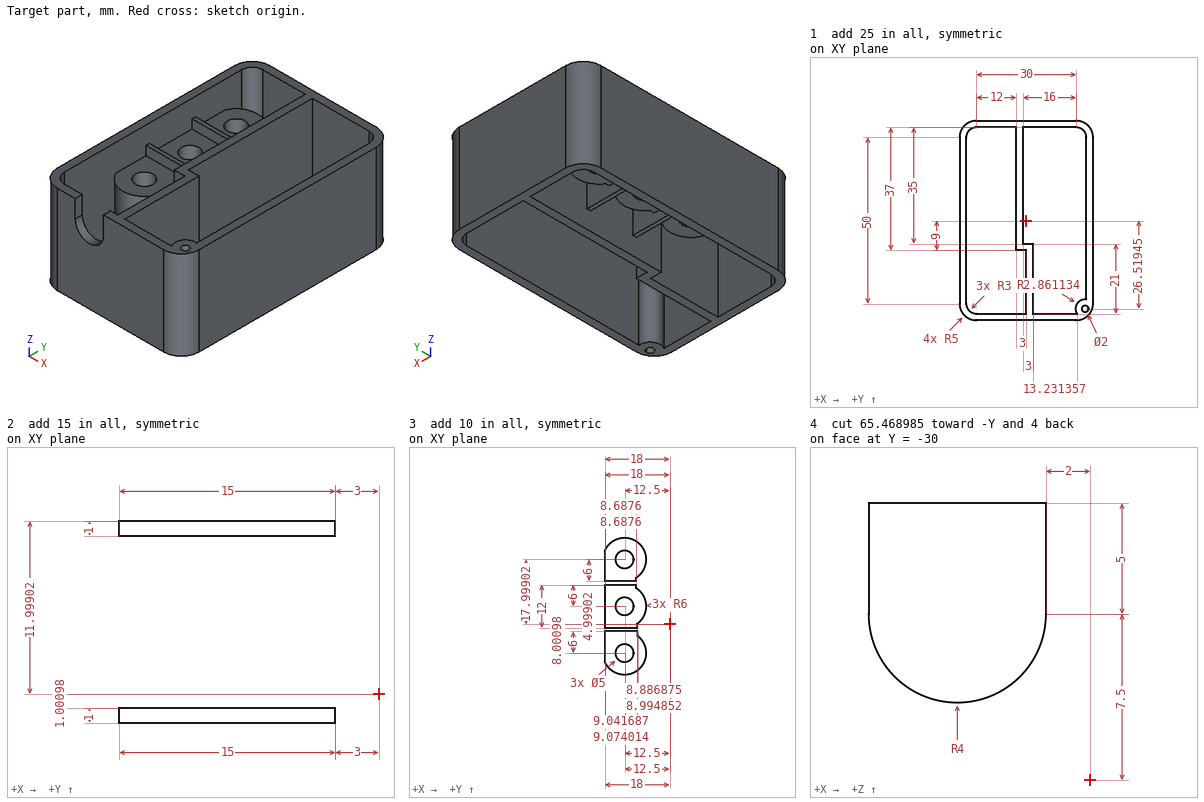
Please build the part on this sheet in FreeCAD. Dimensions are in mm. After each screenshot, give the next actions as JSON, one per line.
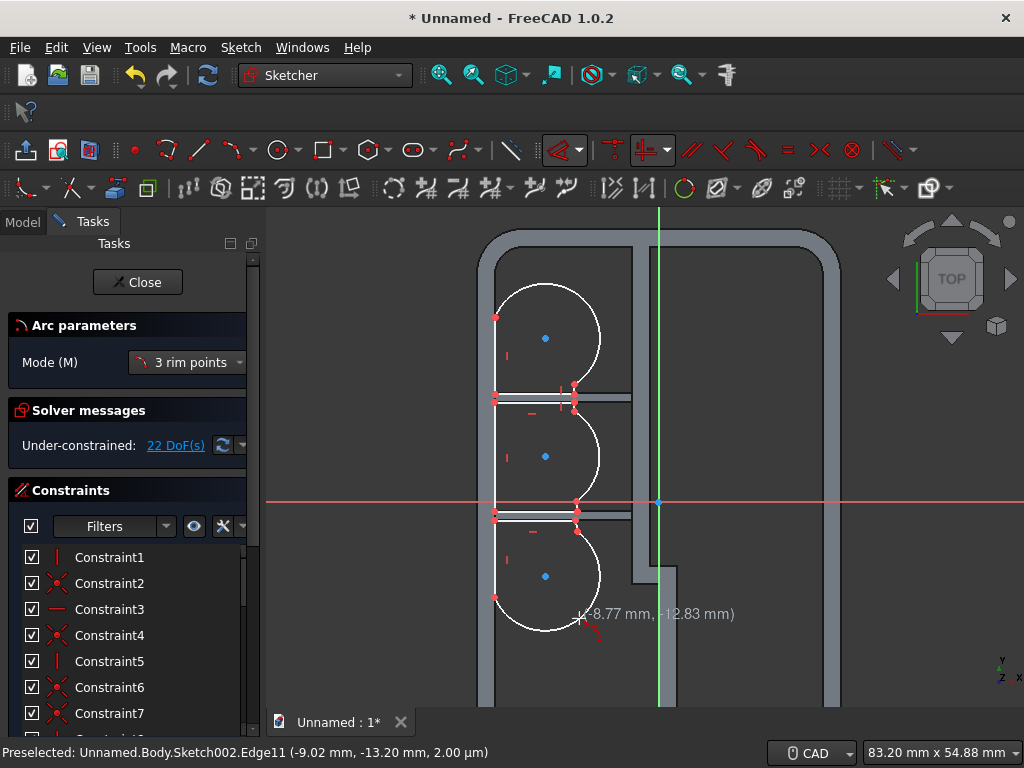
{"action": "left_click", "coordinate": [278, 150]}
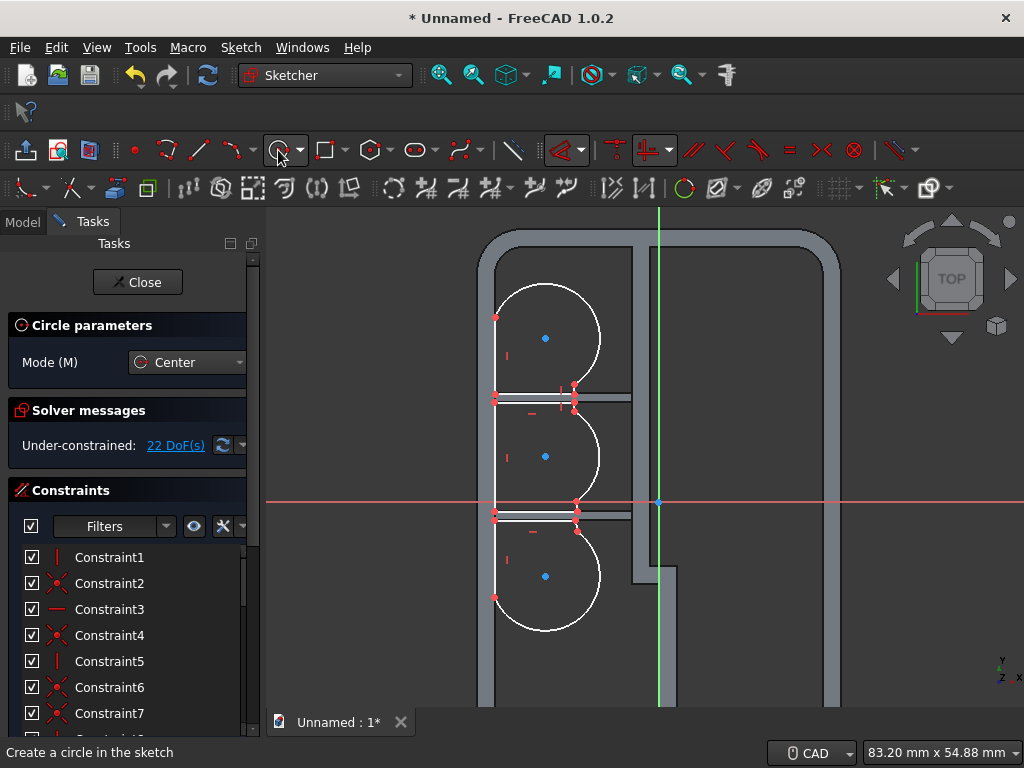
{"action": "left_click", "coordinate": [545, 338]}
{"action": "left_click", "coordinate": [561, 322]}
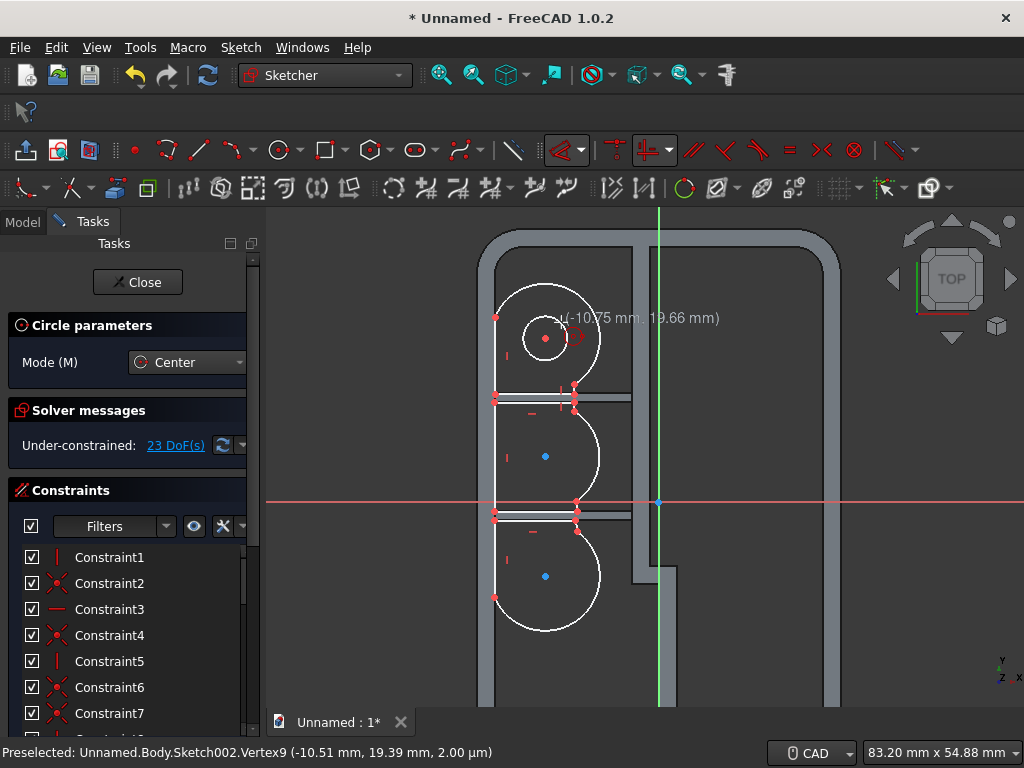
{"action": "left_click", "coordinate": [545, 457]}
{"action": "left_click", "coordinate": [561, 440]}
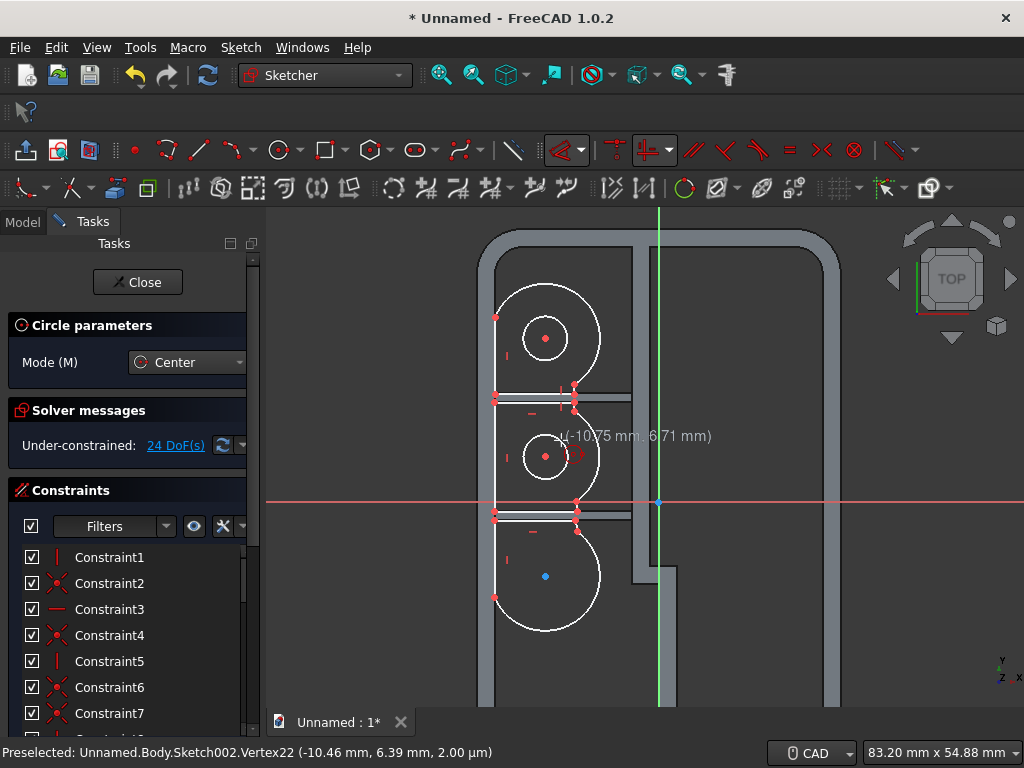
{"action": "left_click", "coordinate": [545, 575]}
{"action": "left_click", "coordinate": [561, 559]}
{"action": "key", "text": "Escape"}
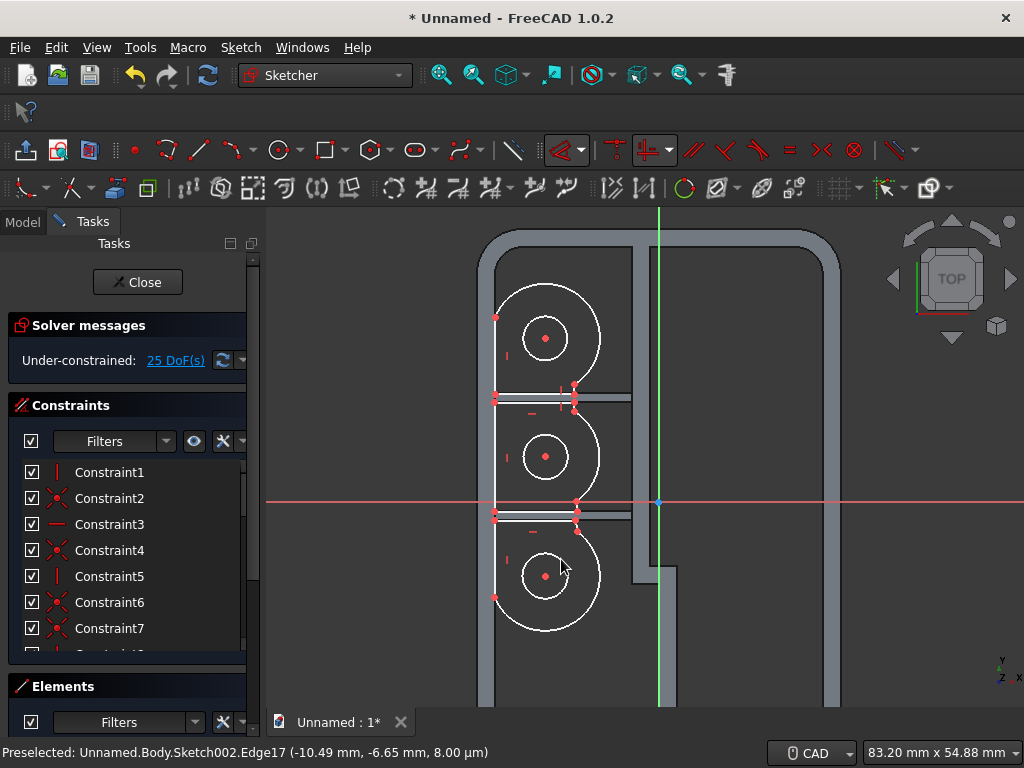
{"action": "left_click", "coordinate": [600, 332]}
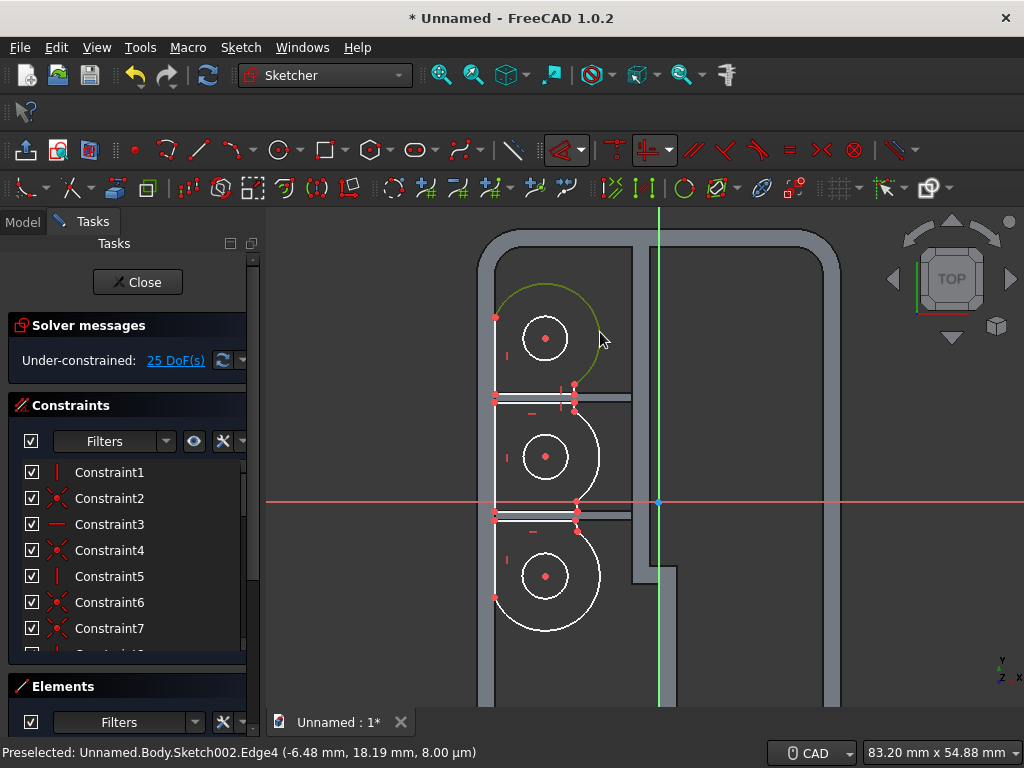
{"action": "left_click", "coordinate": [596, 476]}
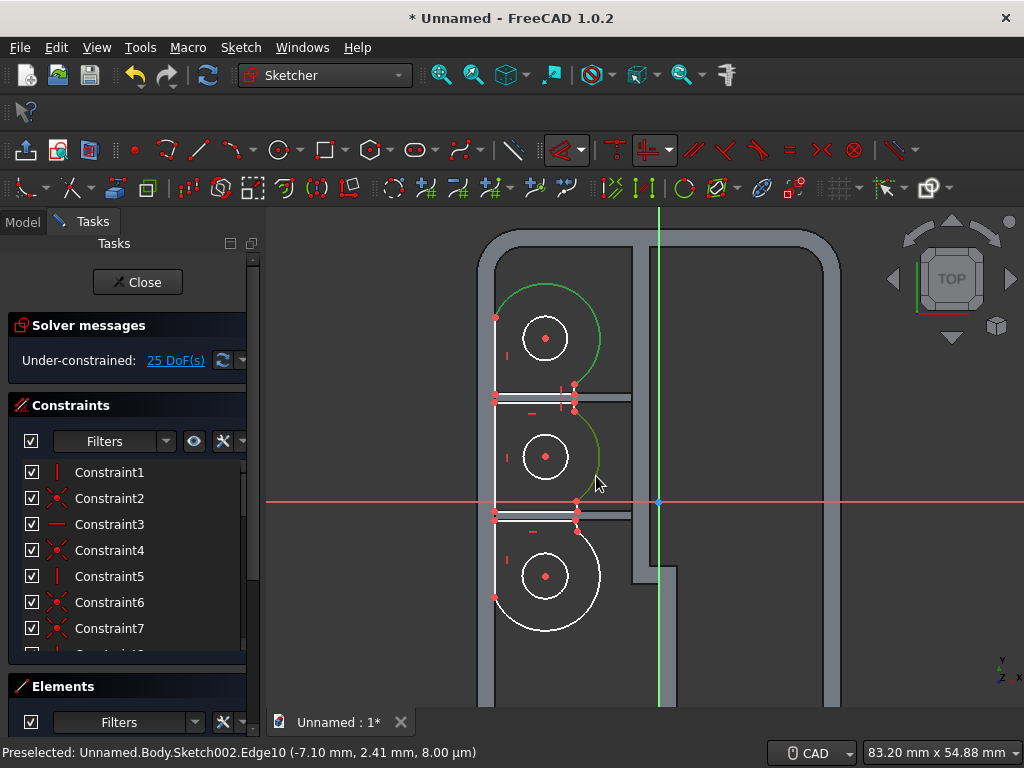
{"action": "left_click", "coordinate": [542, 631]}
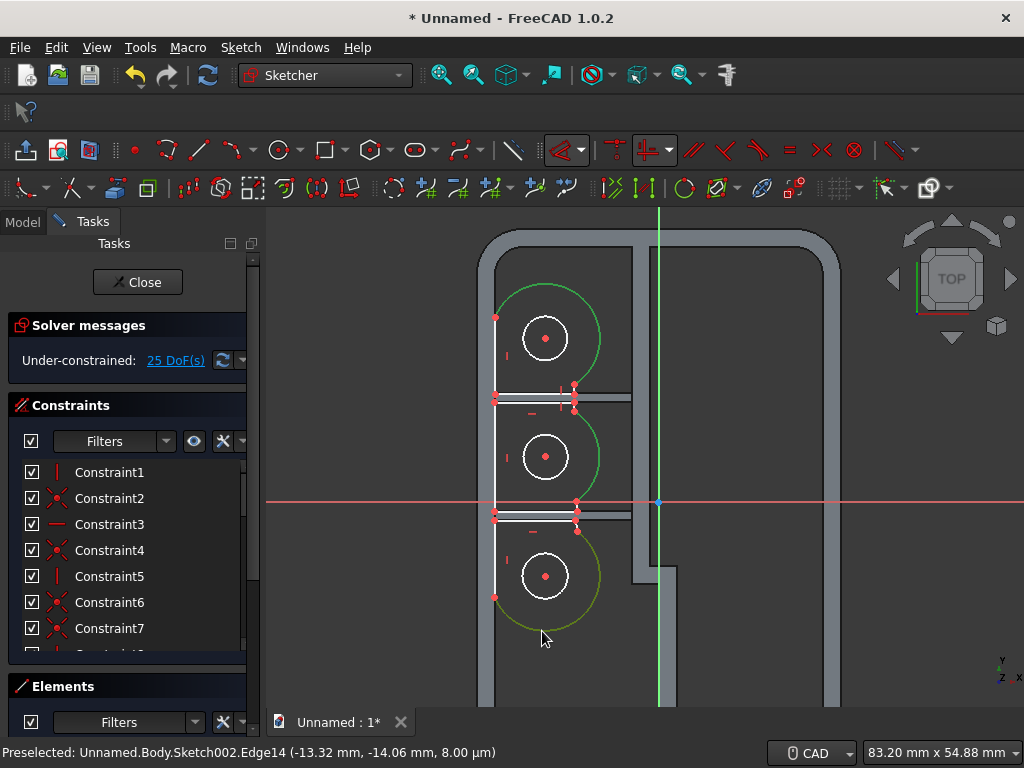
{"action": "left_click", "coordinate": [790, 150]}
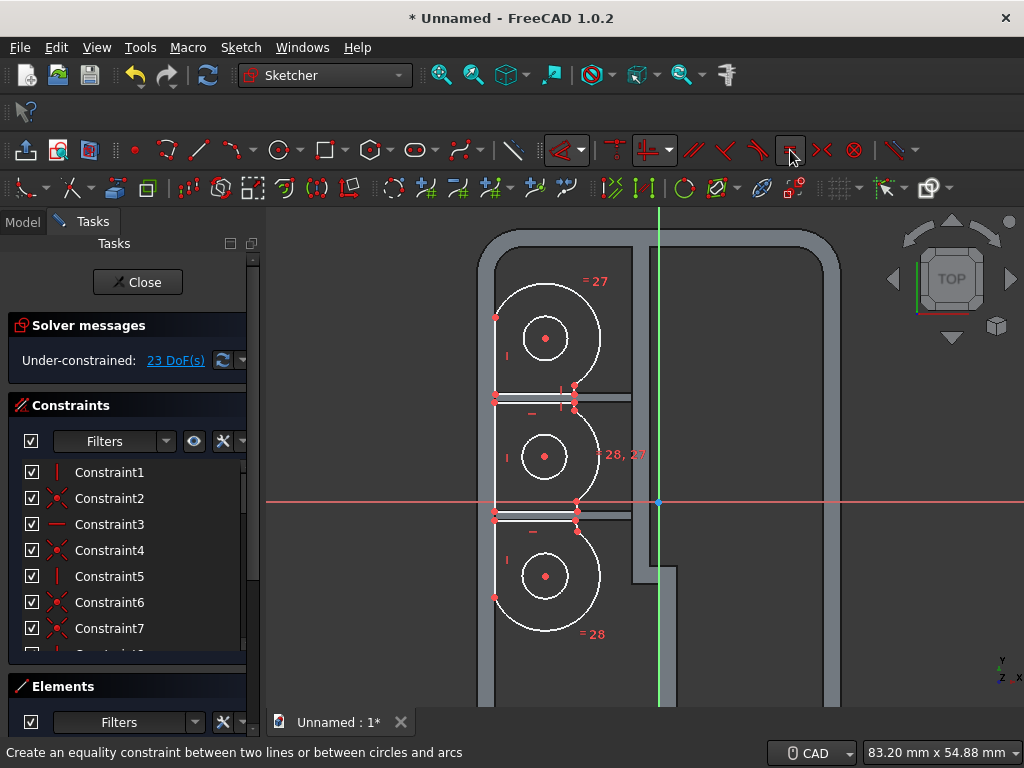
{"action": "left_click", "coordinate": [561, 323]}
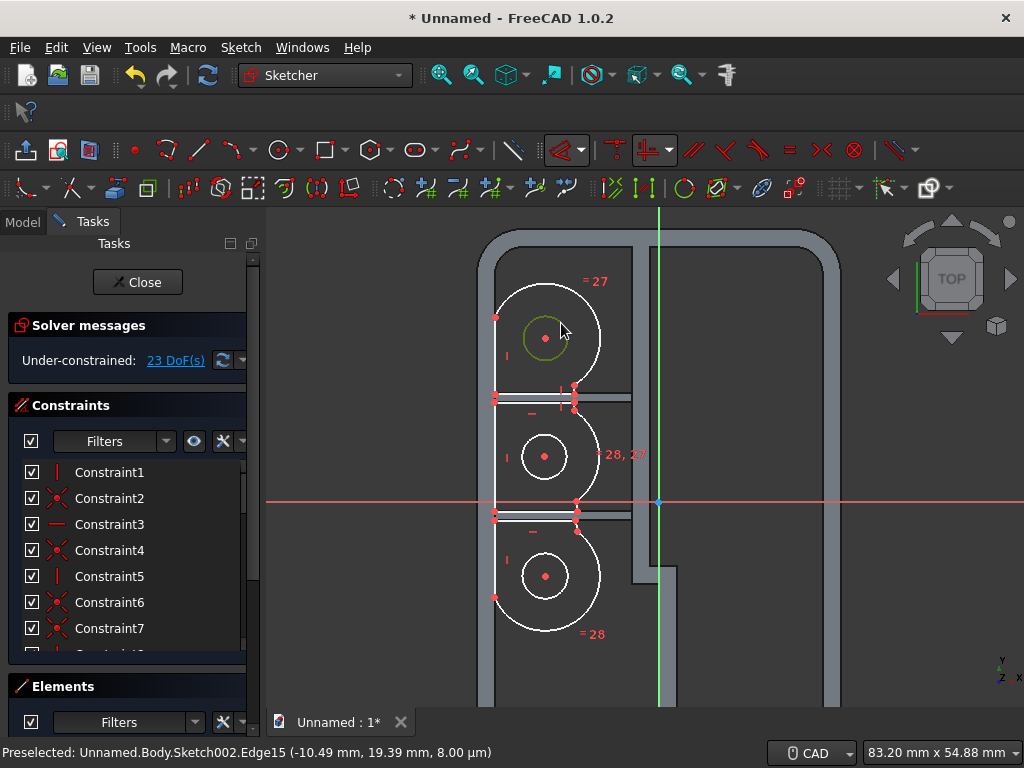
{"action": "left_click", "coordinate": [560, 441]}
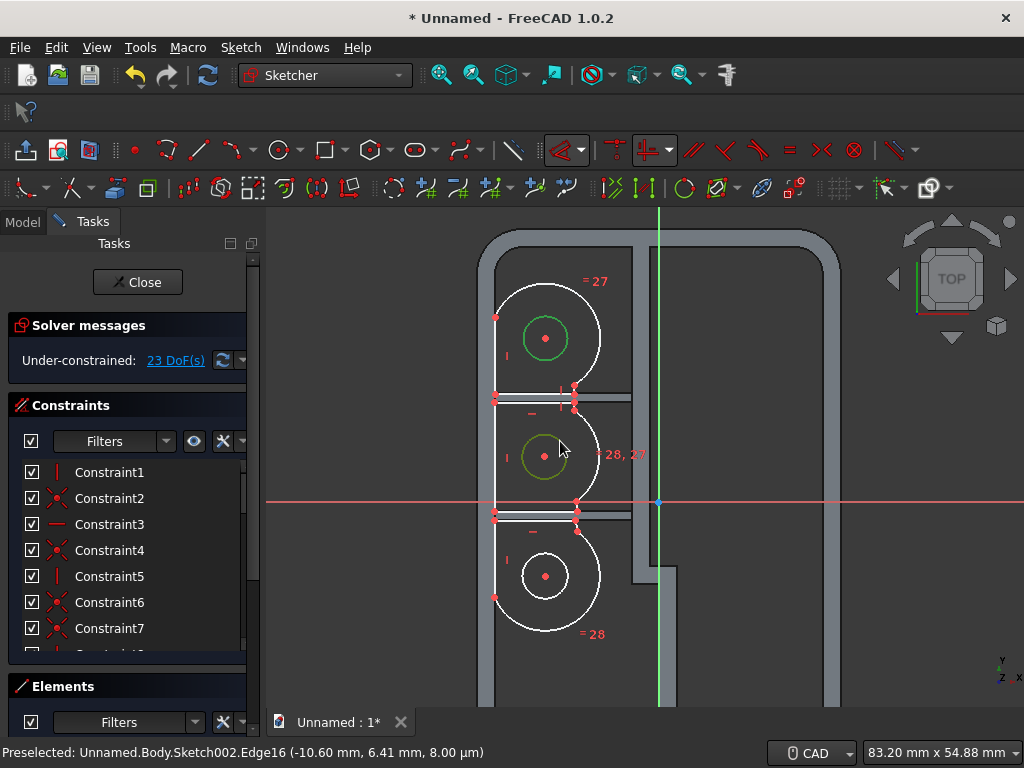
{"action": "left_click", "coordinate": [561, 560]}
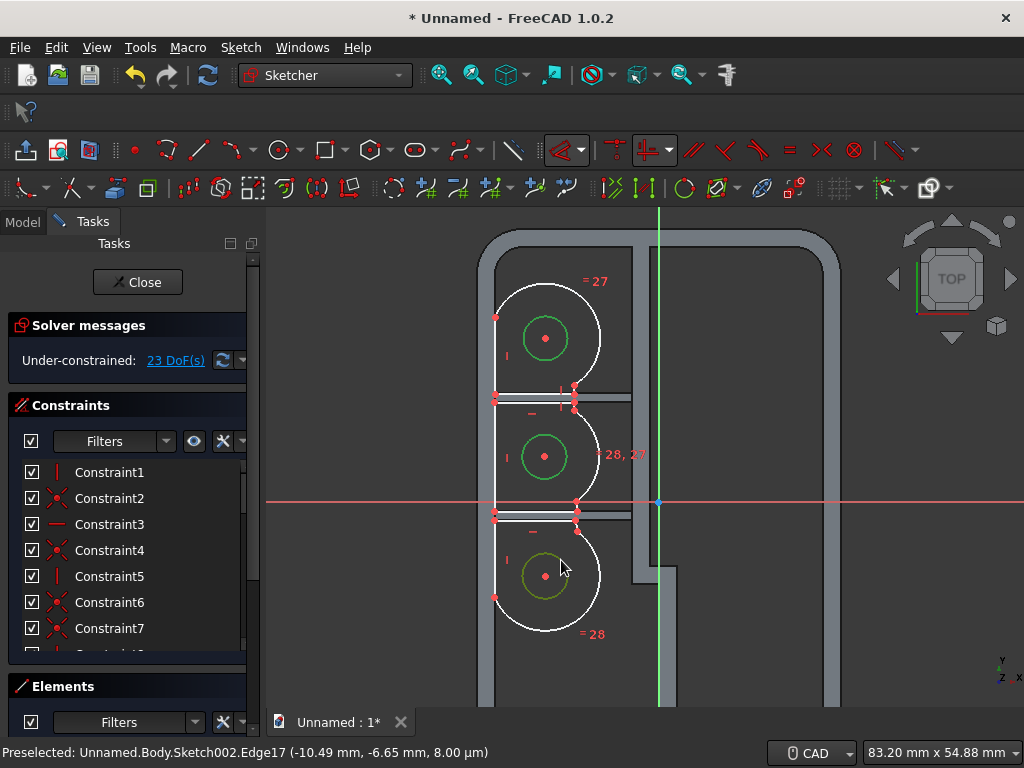
{"action": "left_click", "coordinate": [790, 150]}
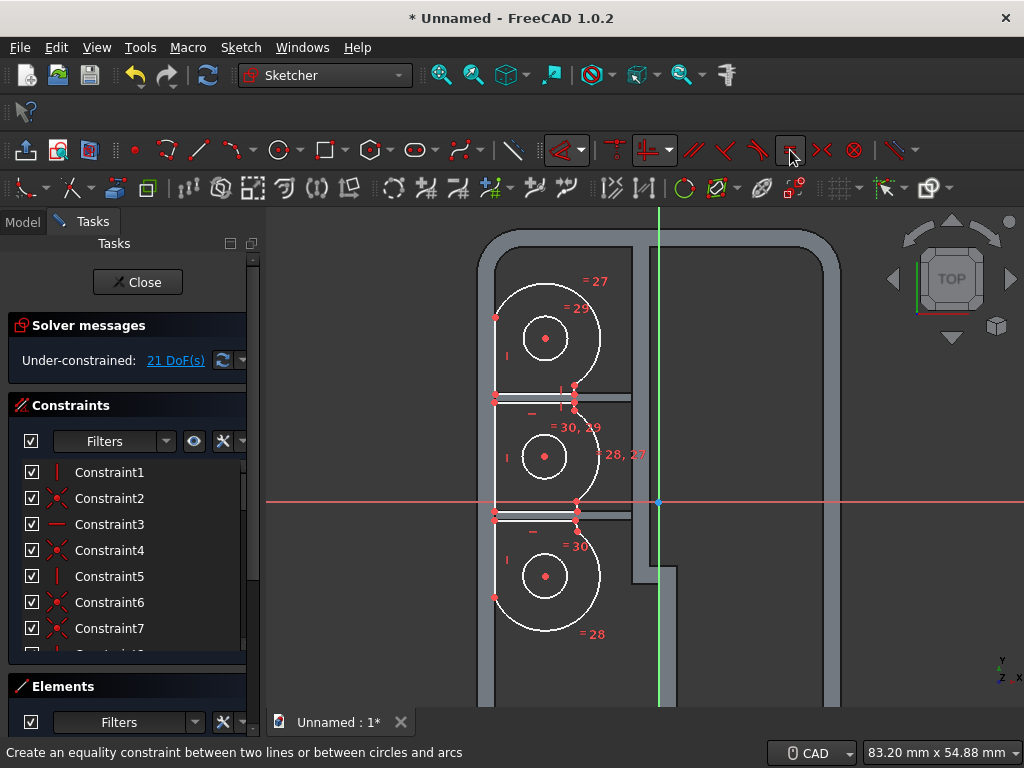
{"action": "left_click", "coordinate": [600, 333]}